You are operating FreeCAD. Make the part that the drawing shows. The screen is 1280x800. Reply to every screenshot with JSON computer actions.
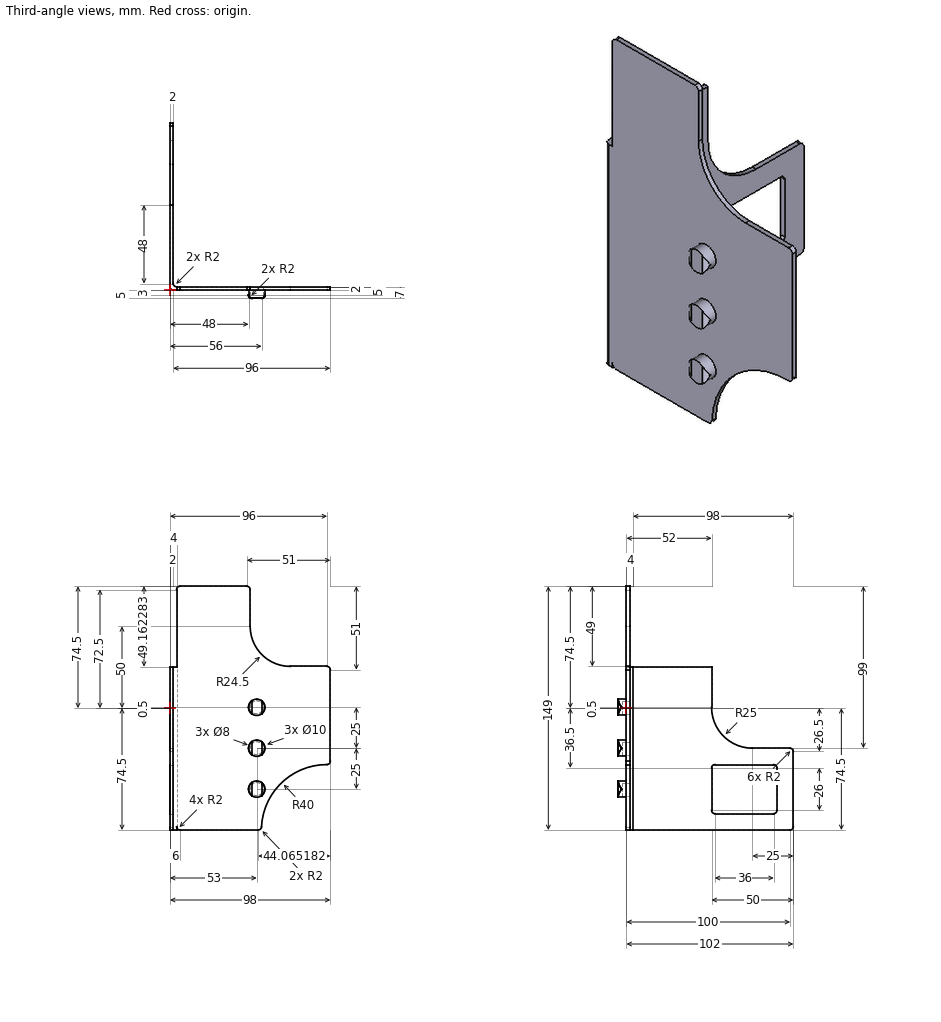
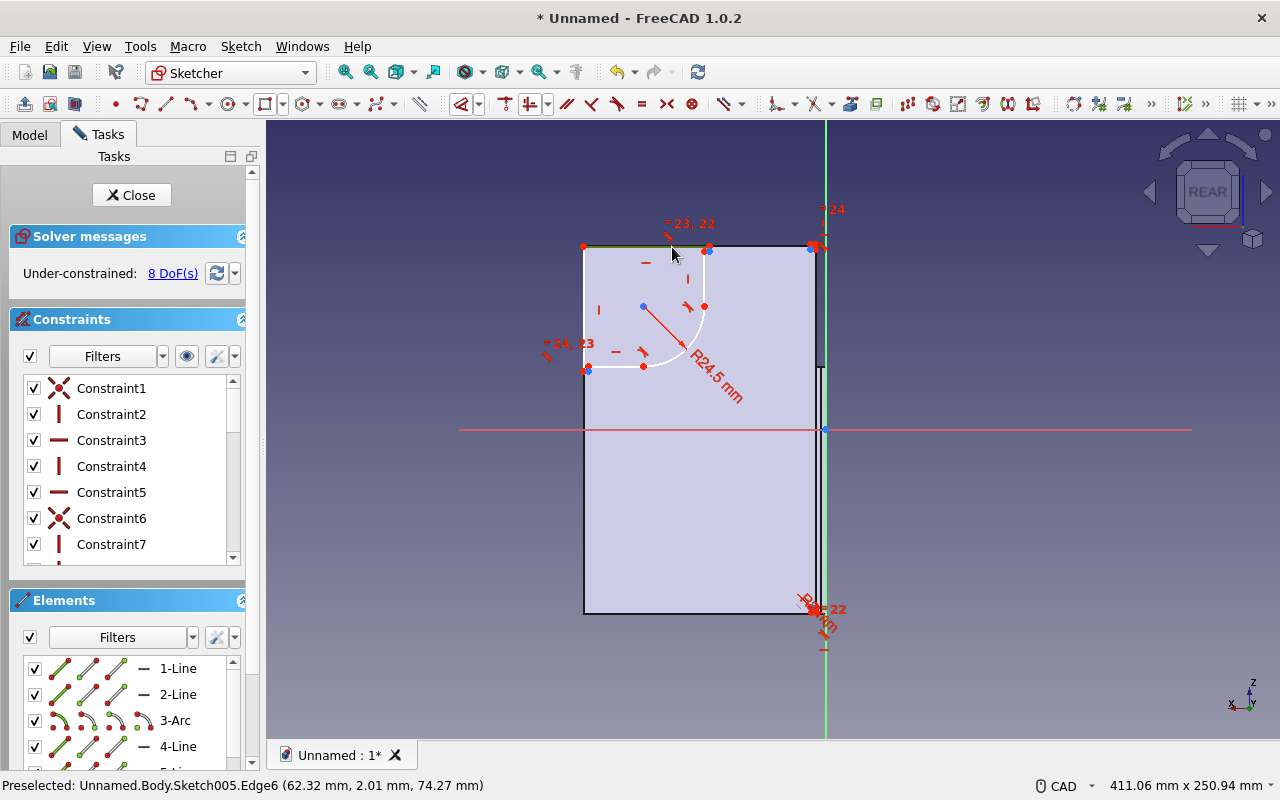
{"action": "key", "text": "l"}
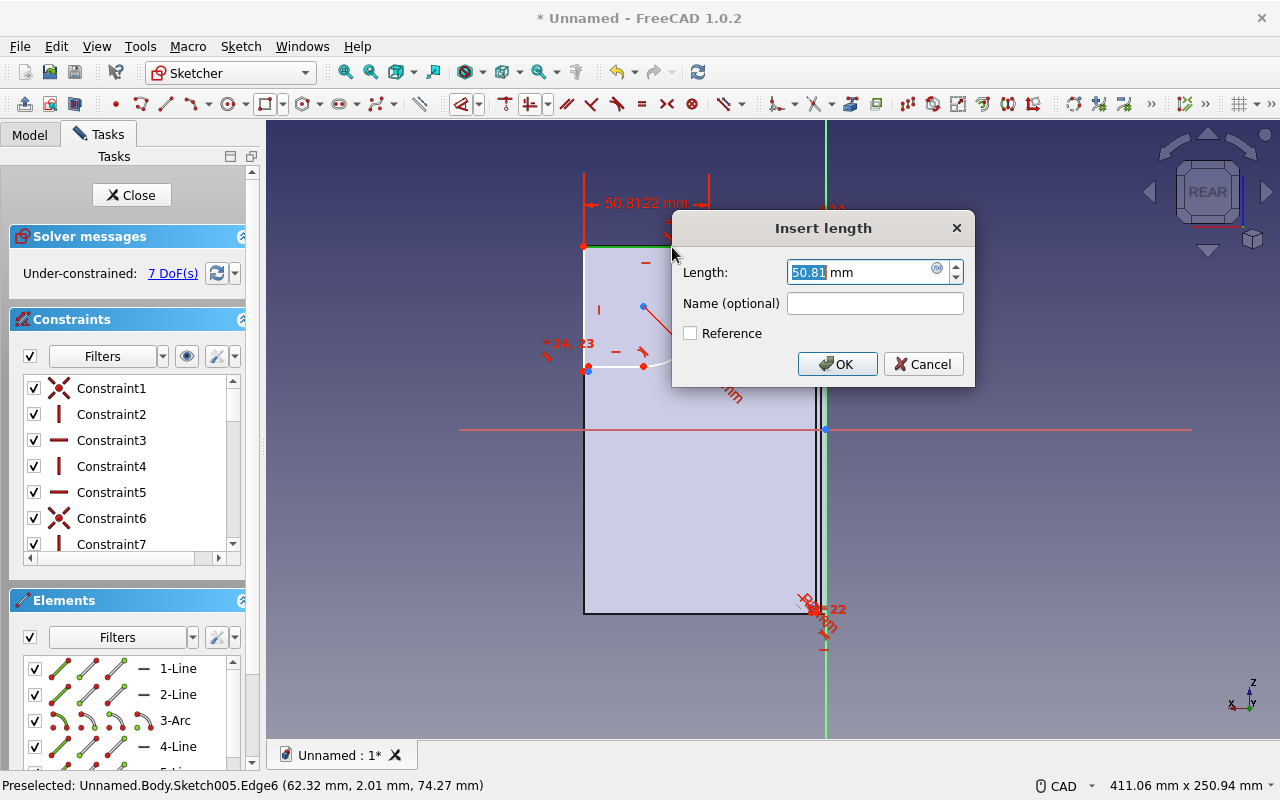
{"action": "type", "text": "51"}
{"action": "key", "text": "Return"}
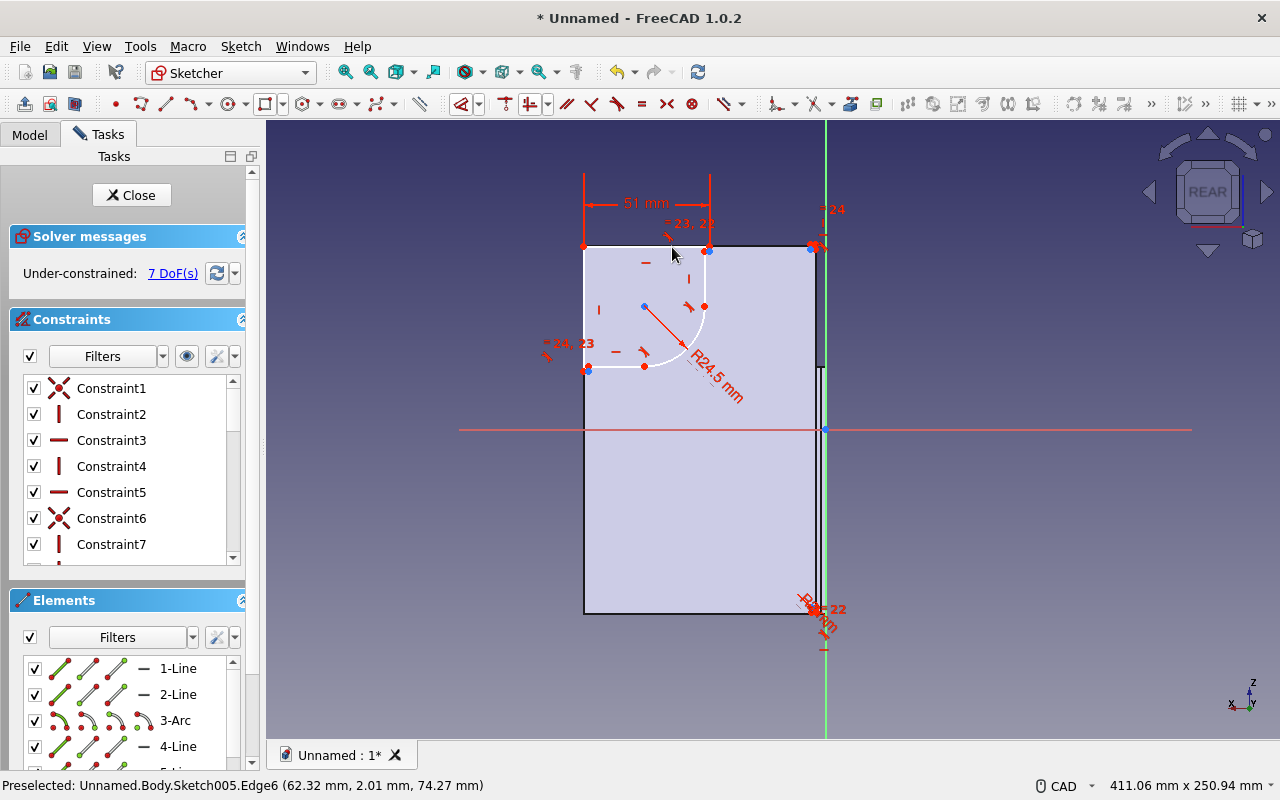
{"action": "left_click", "coordinate": [584, 284]}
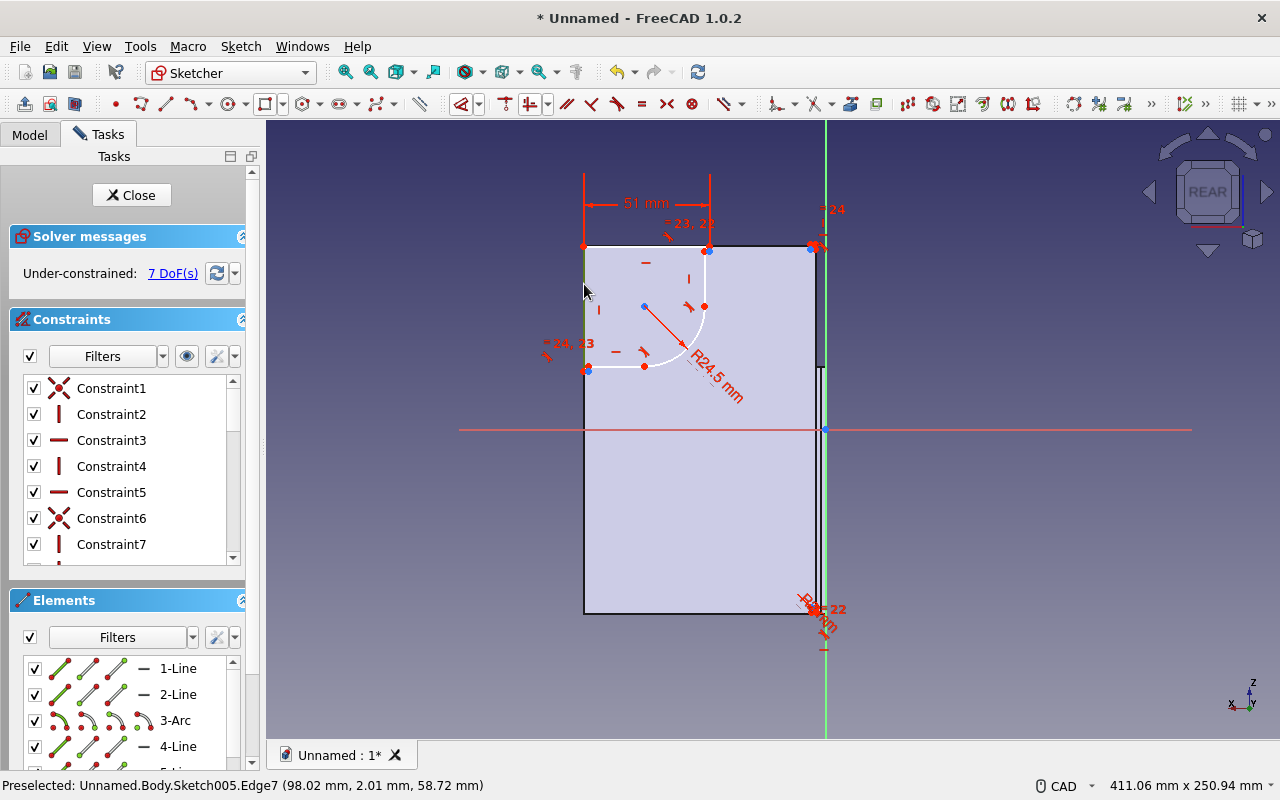
{"action": "key", "text": "i"}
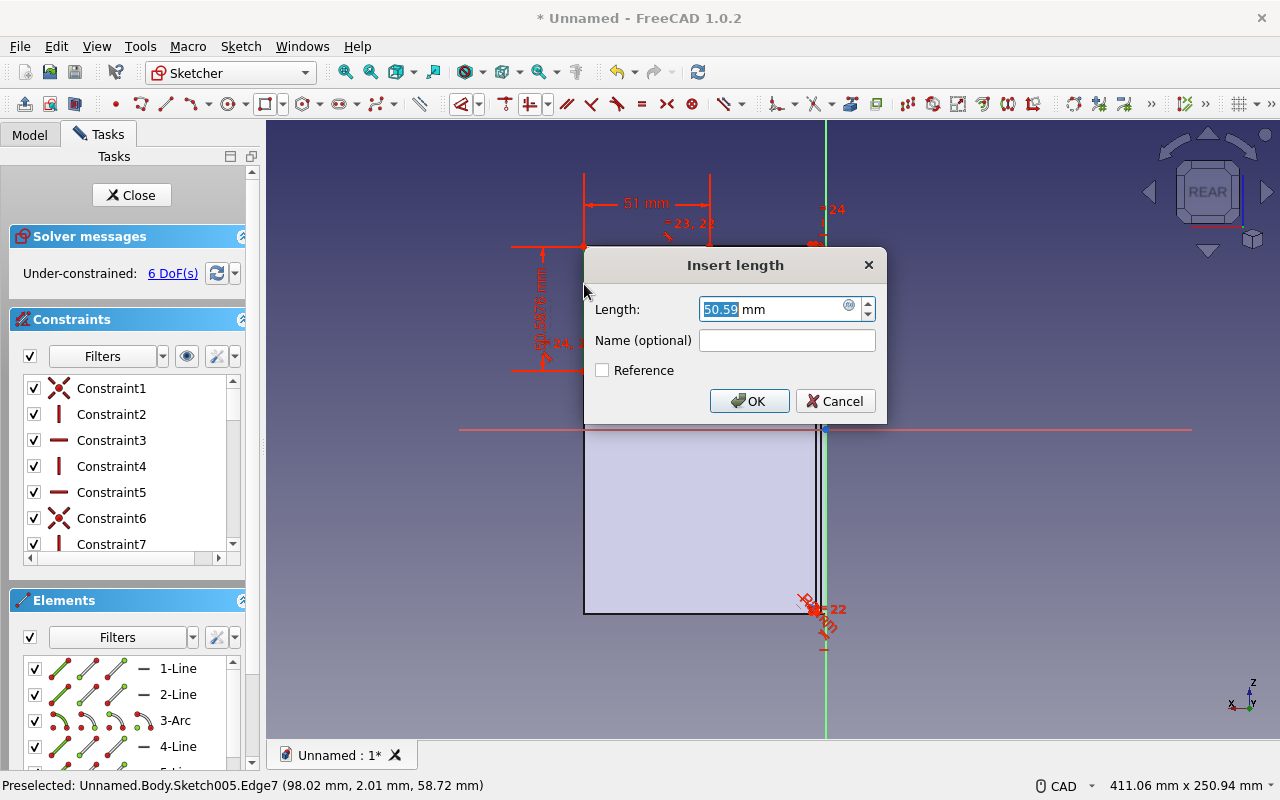
{"action": "type", "text": "51"}
{"action": "key", "text": "Return"}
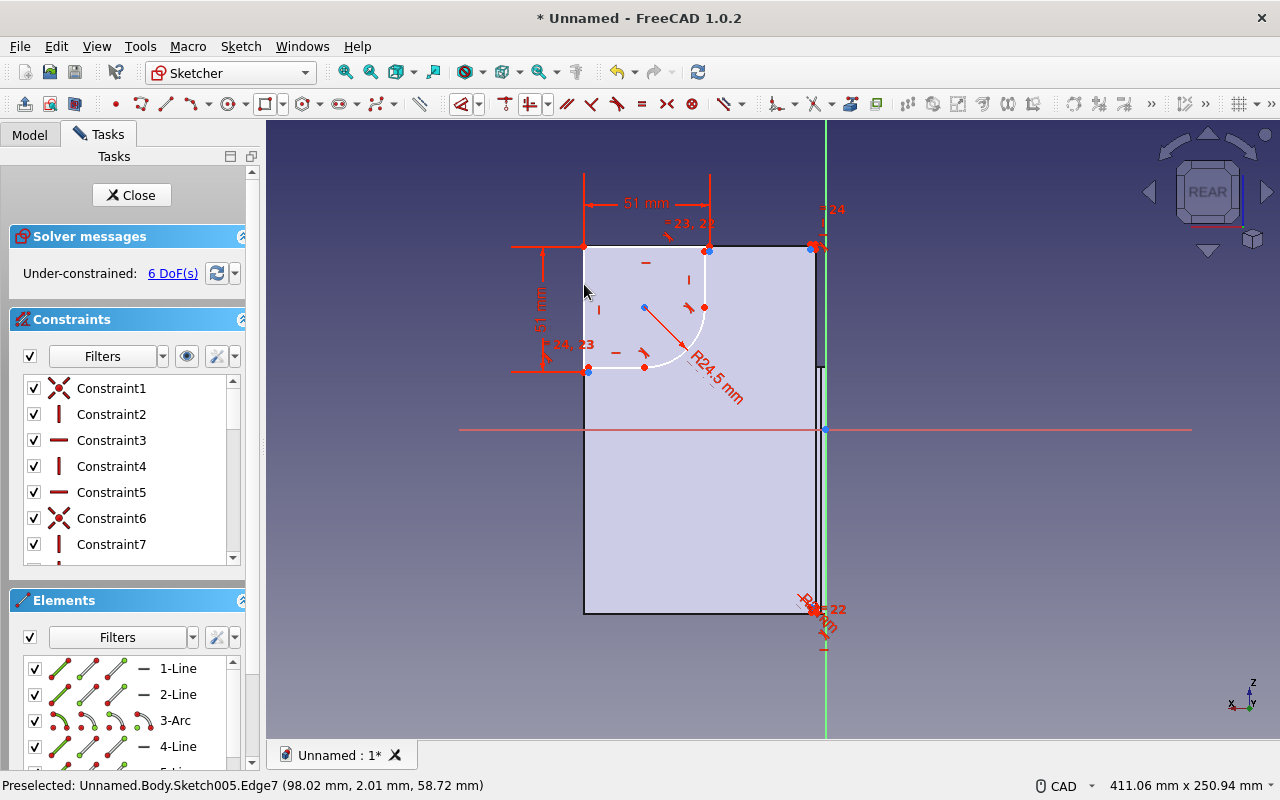
{"action": "scroll", "coordinate": [811, 613], "scroll_direction": "up", "scroll_amount": 5}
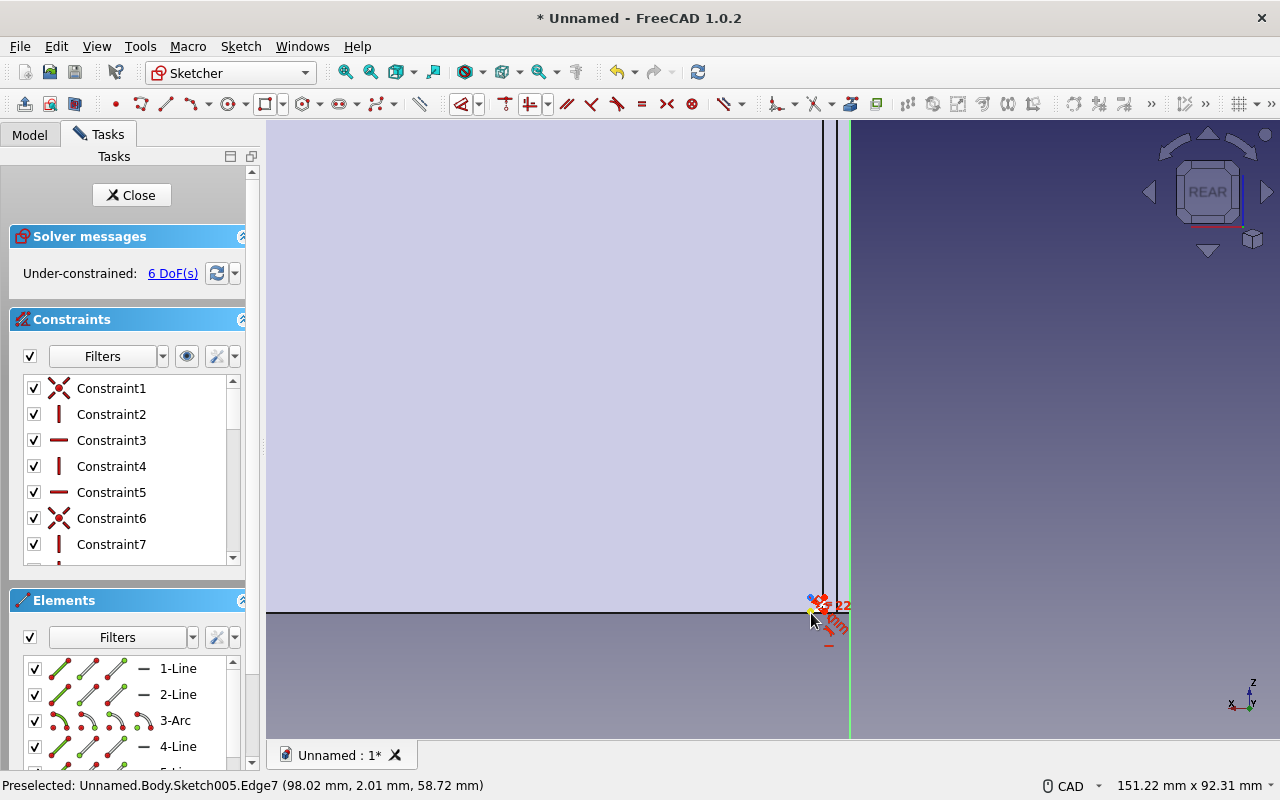
{"action": "left_click", "coordinate": [811, 611]}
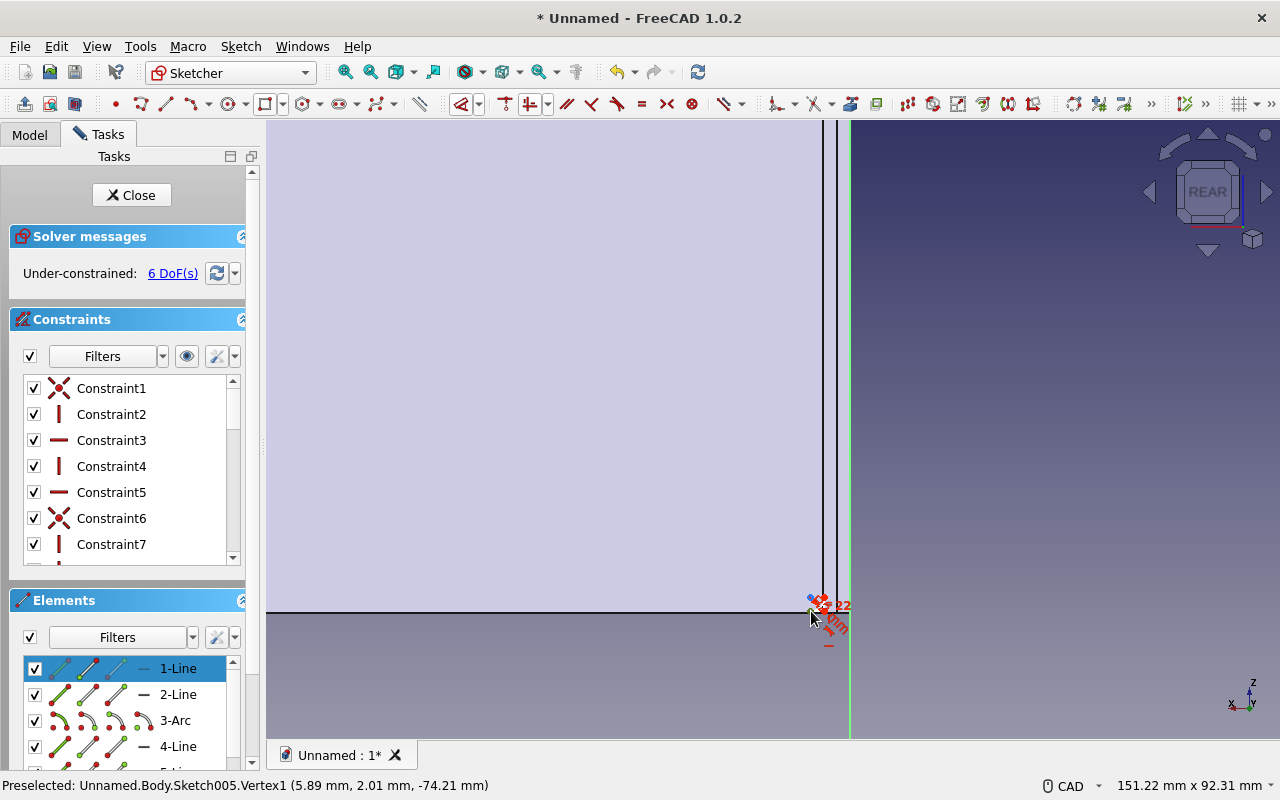
{"action": "left_click", "coordinate": [478, 104]}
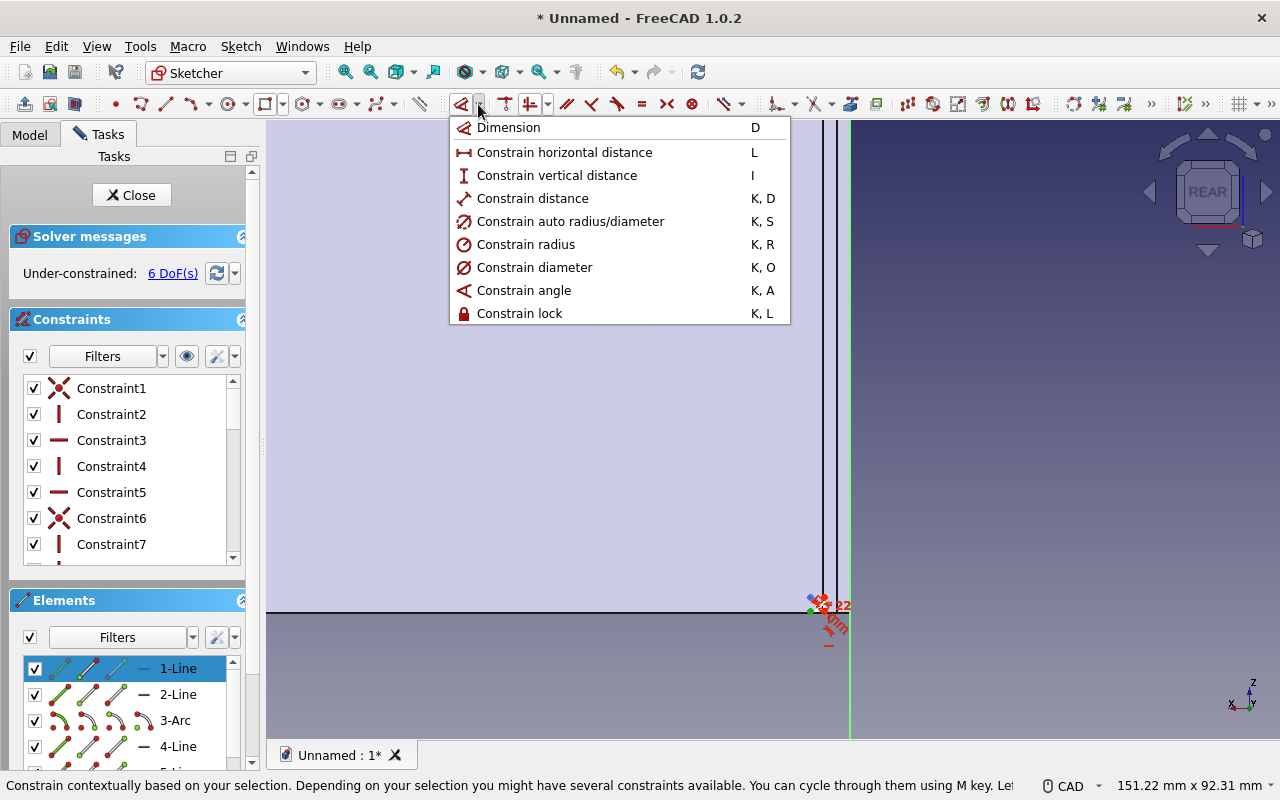
{"action": "left_click", "coordinate": [620, 152]}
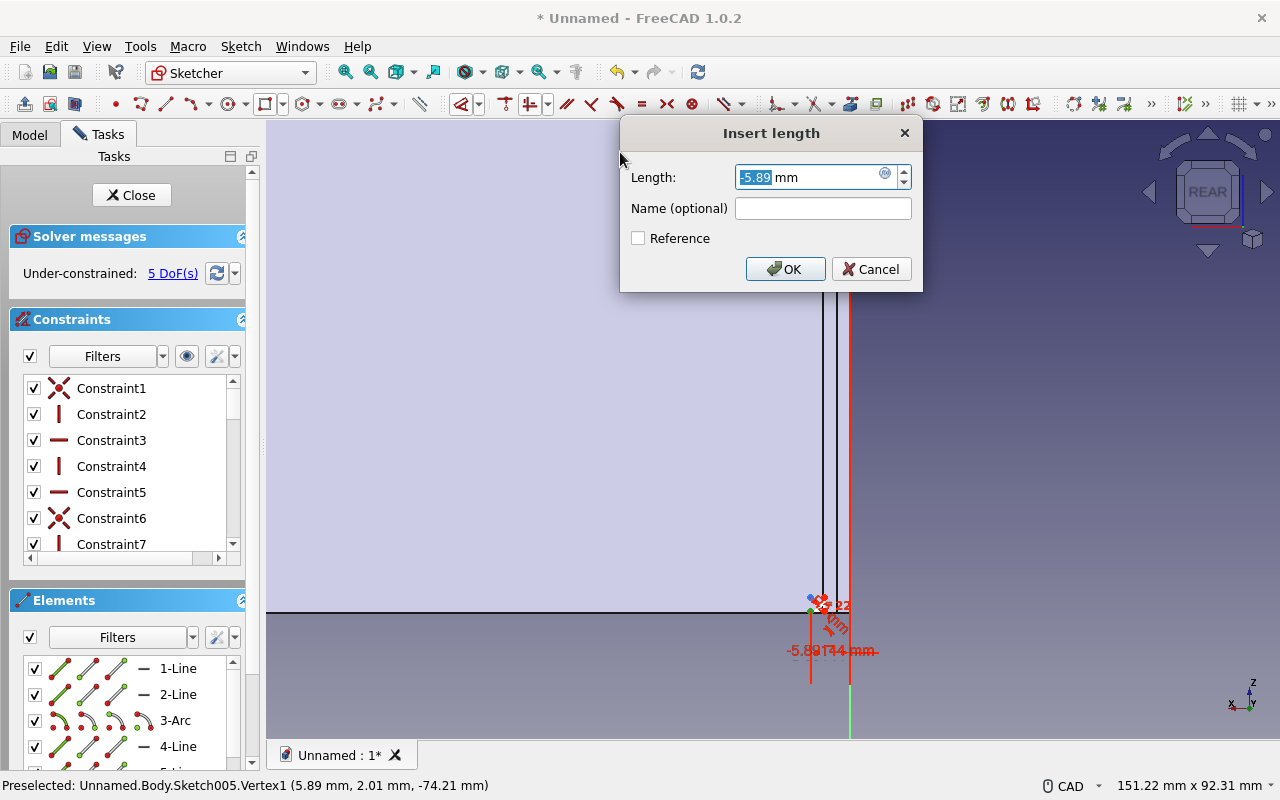
{"action": "type", "text": "-6"}
{"action": "key", "text": "Return"}